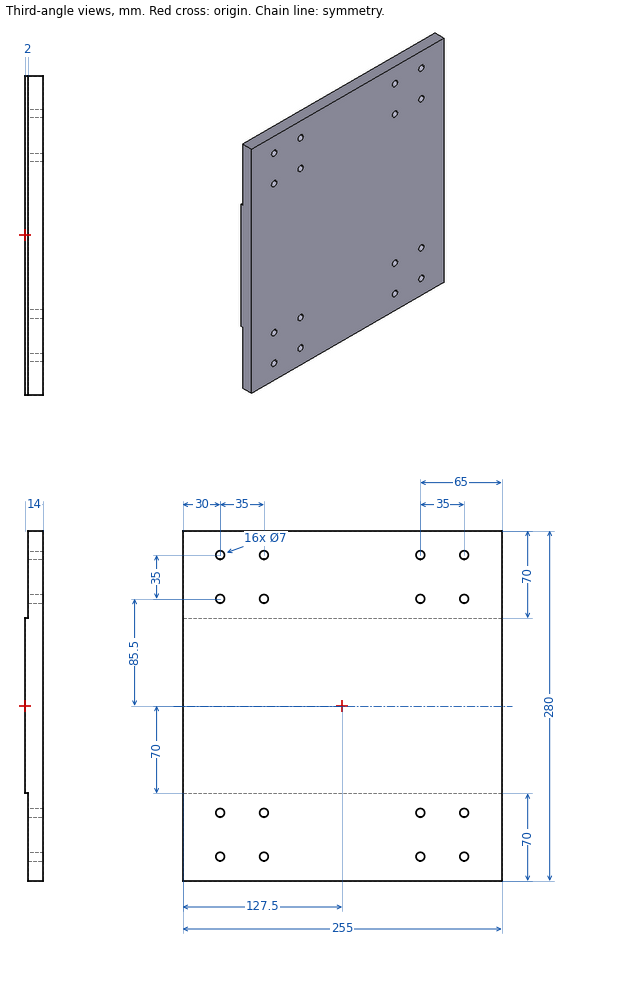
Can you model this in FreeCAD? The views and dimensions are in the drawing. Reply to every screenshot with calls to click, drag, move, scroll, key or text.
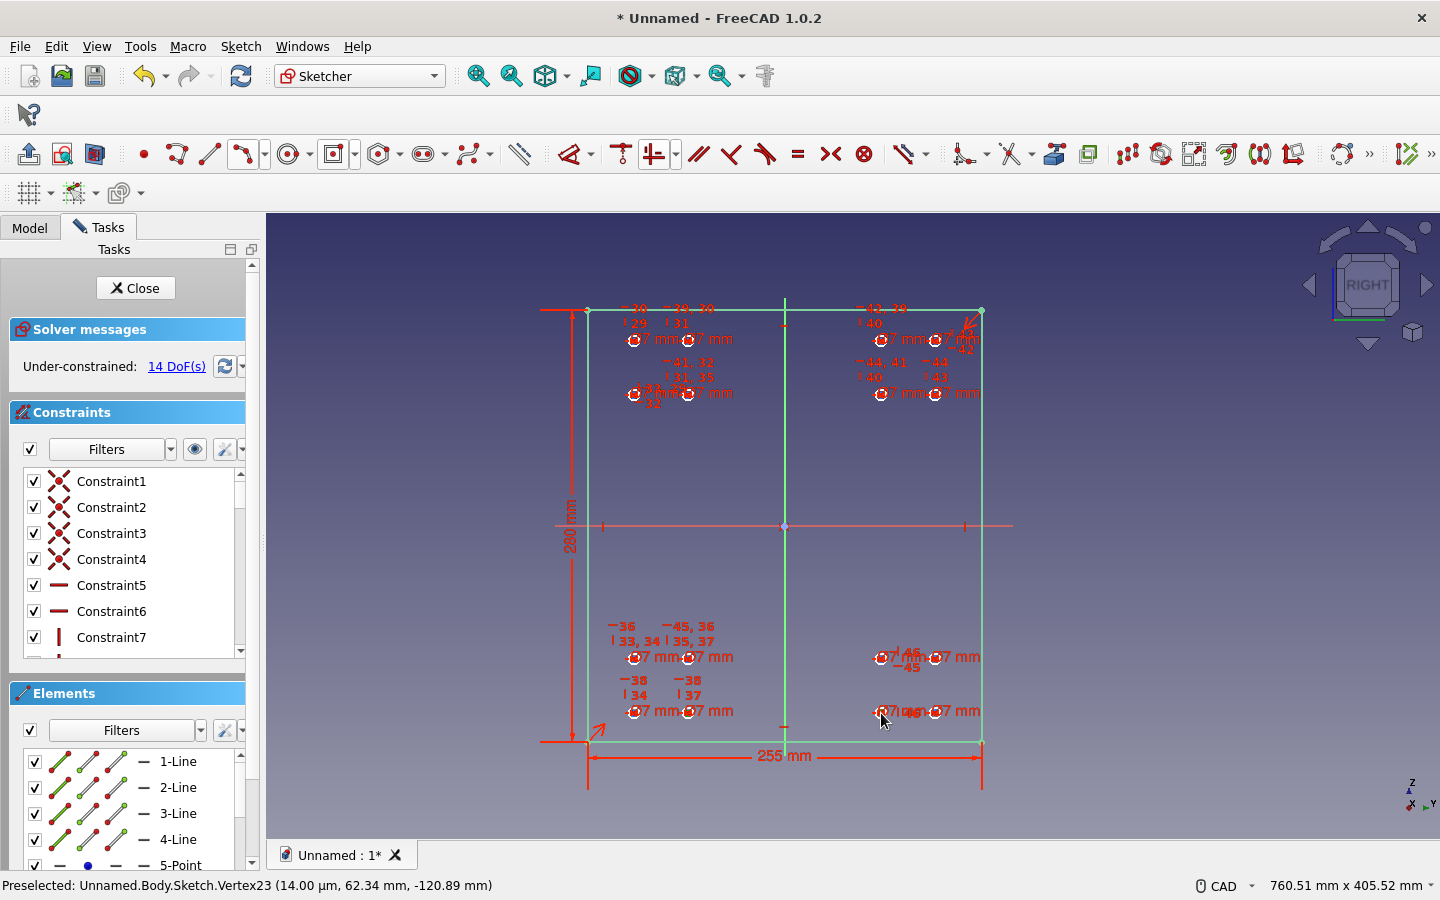
key(h)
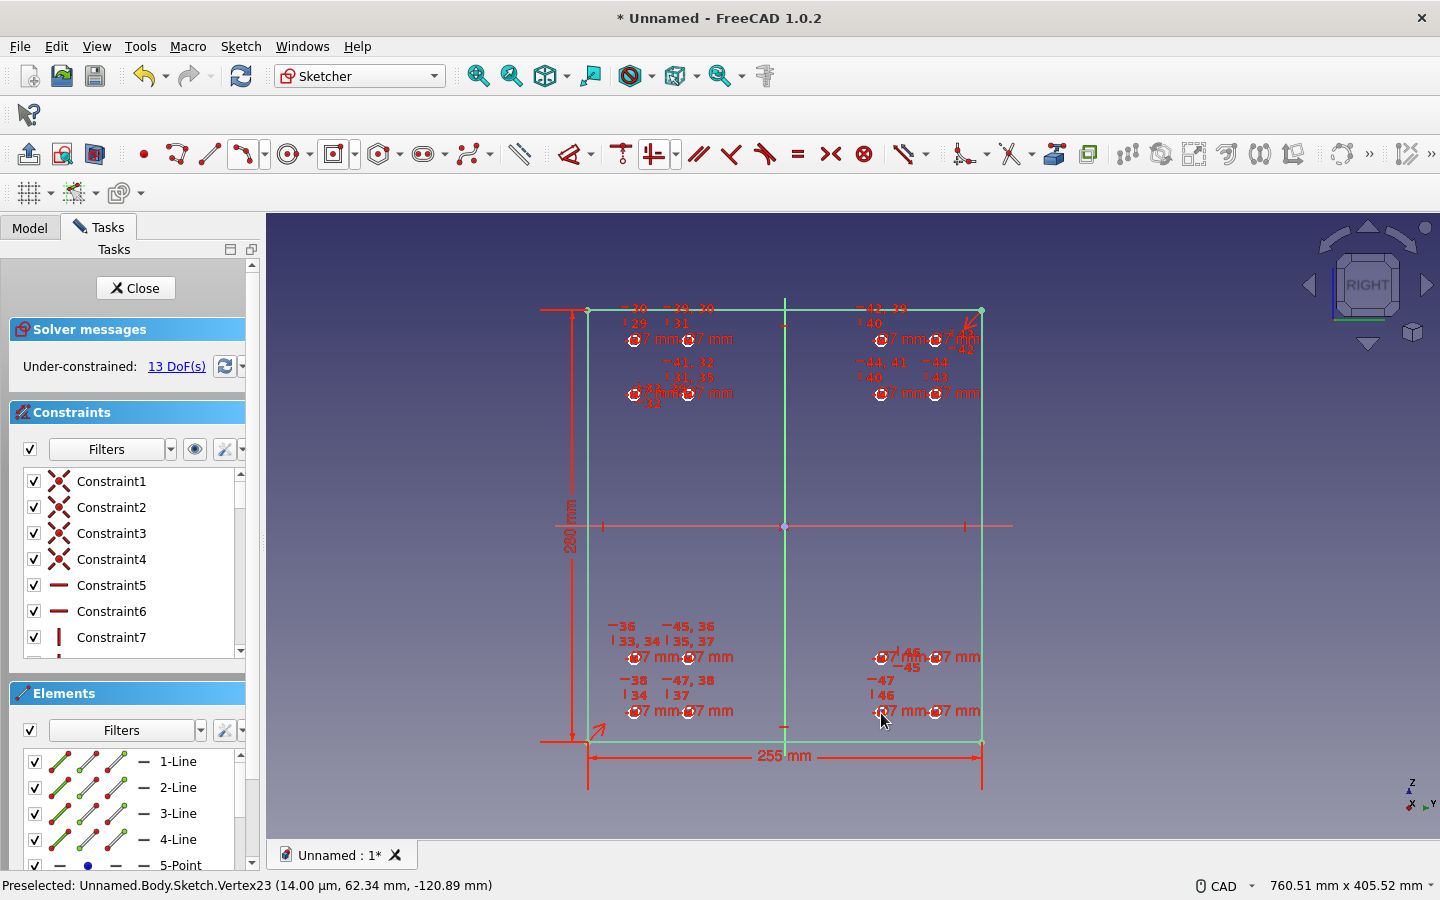
click(881, 659)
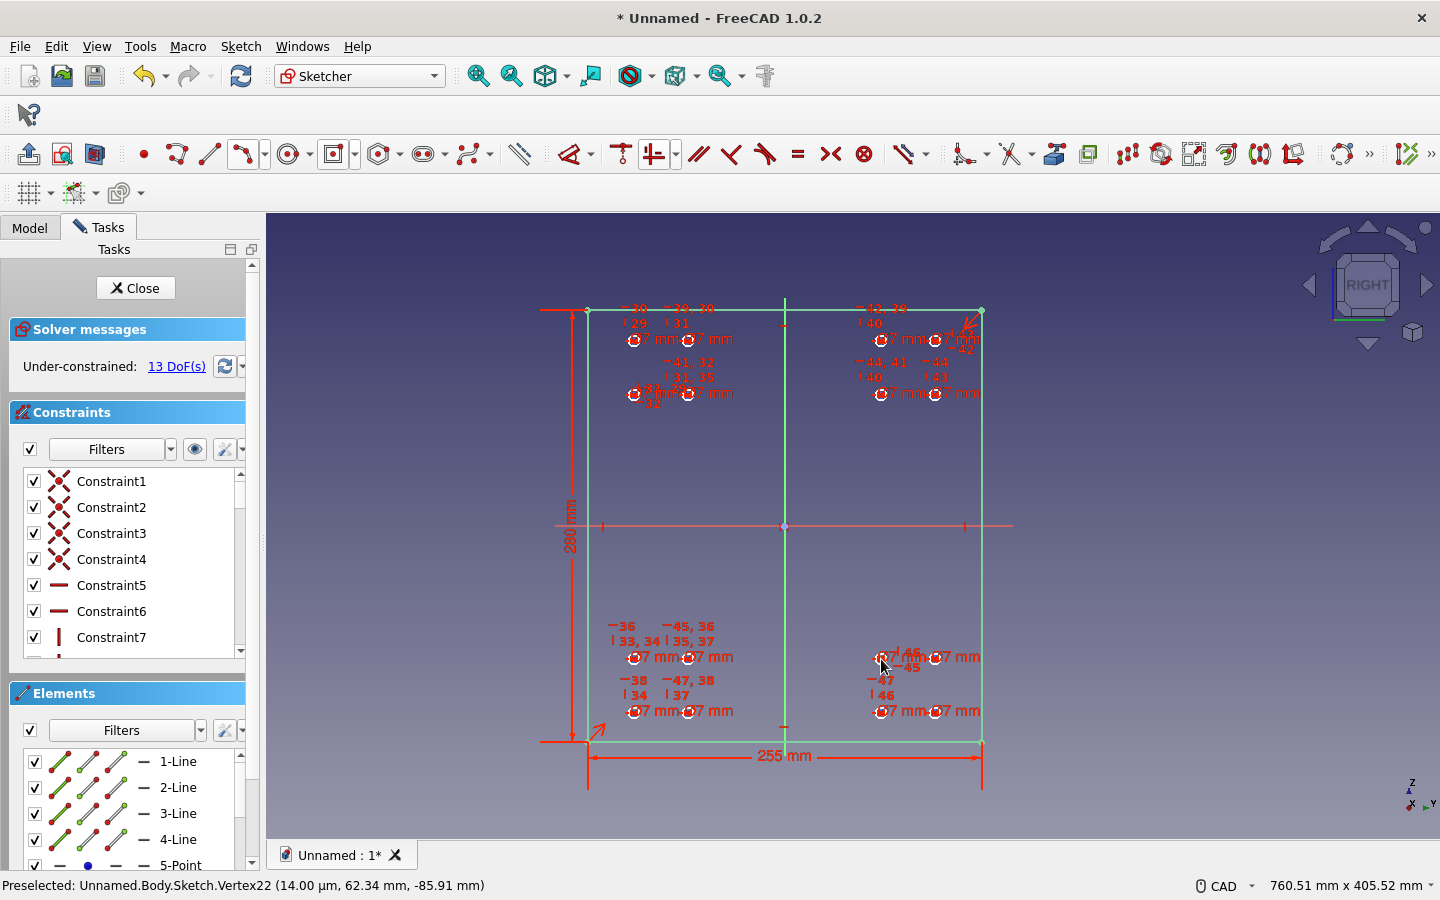
click(935, 659)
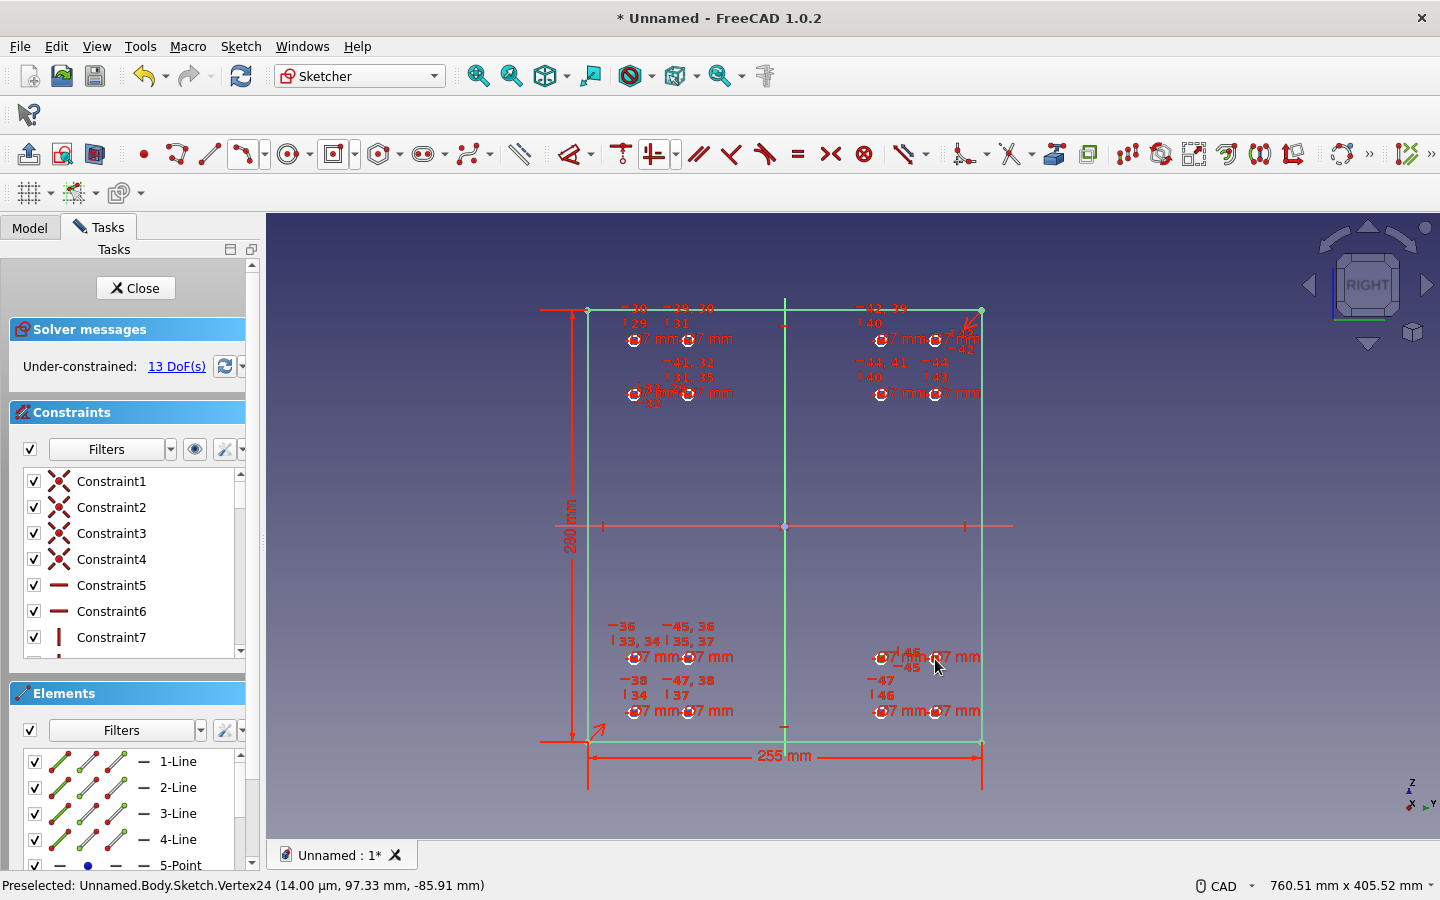
key(h)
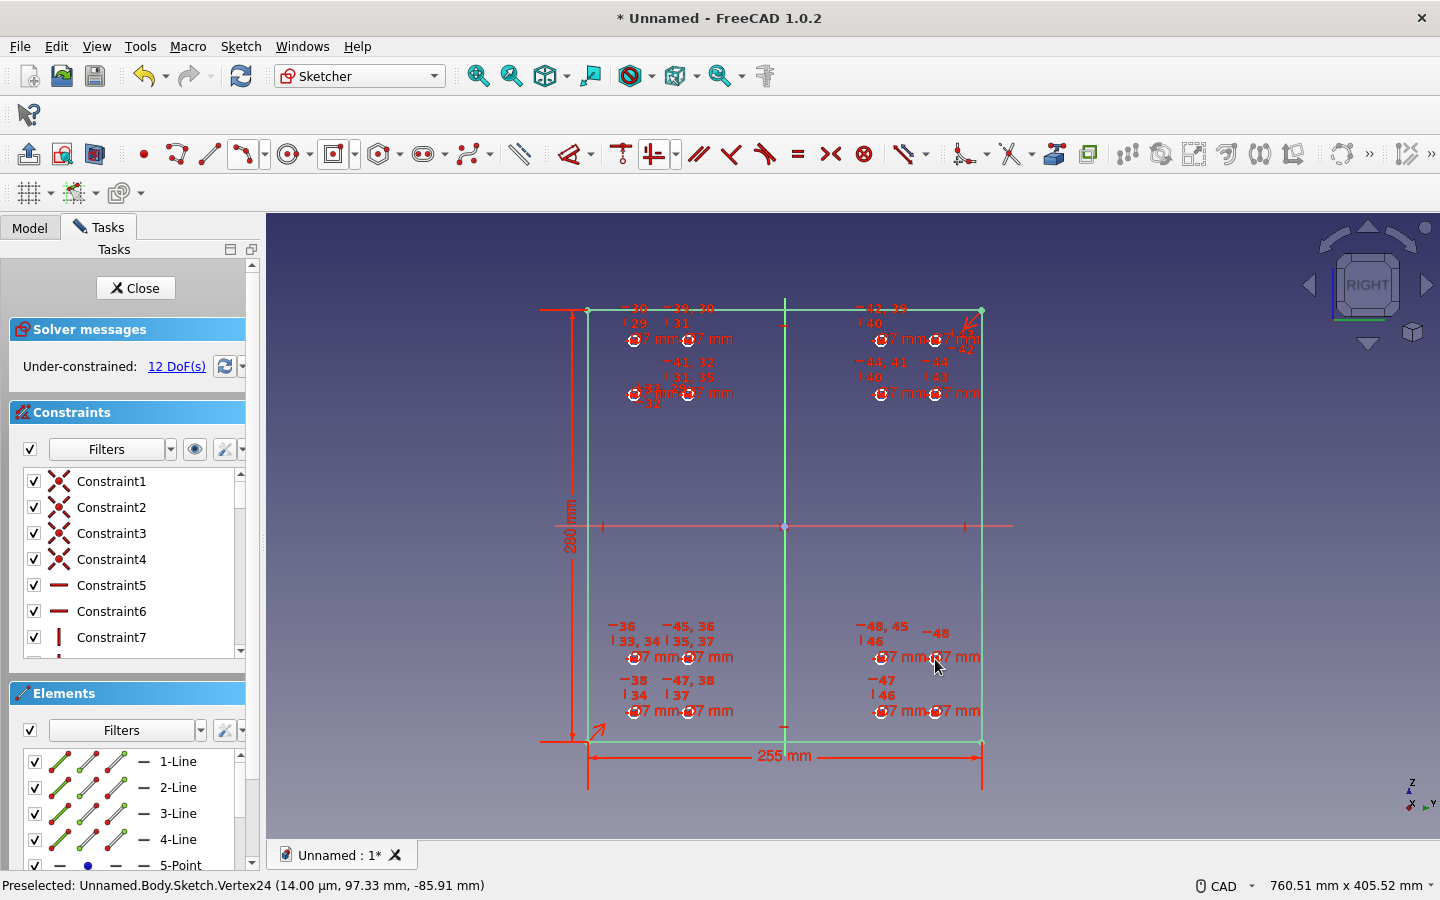
click(935, 659)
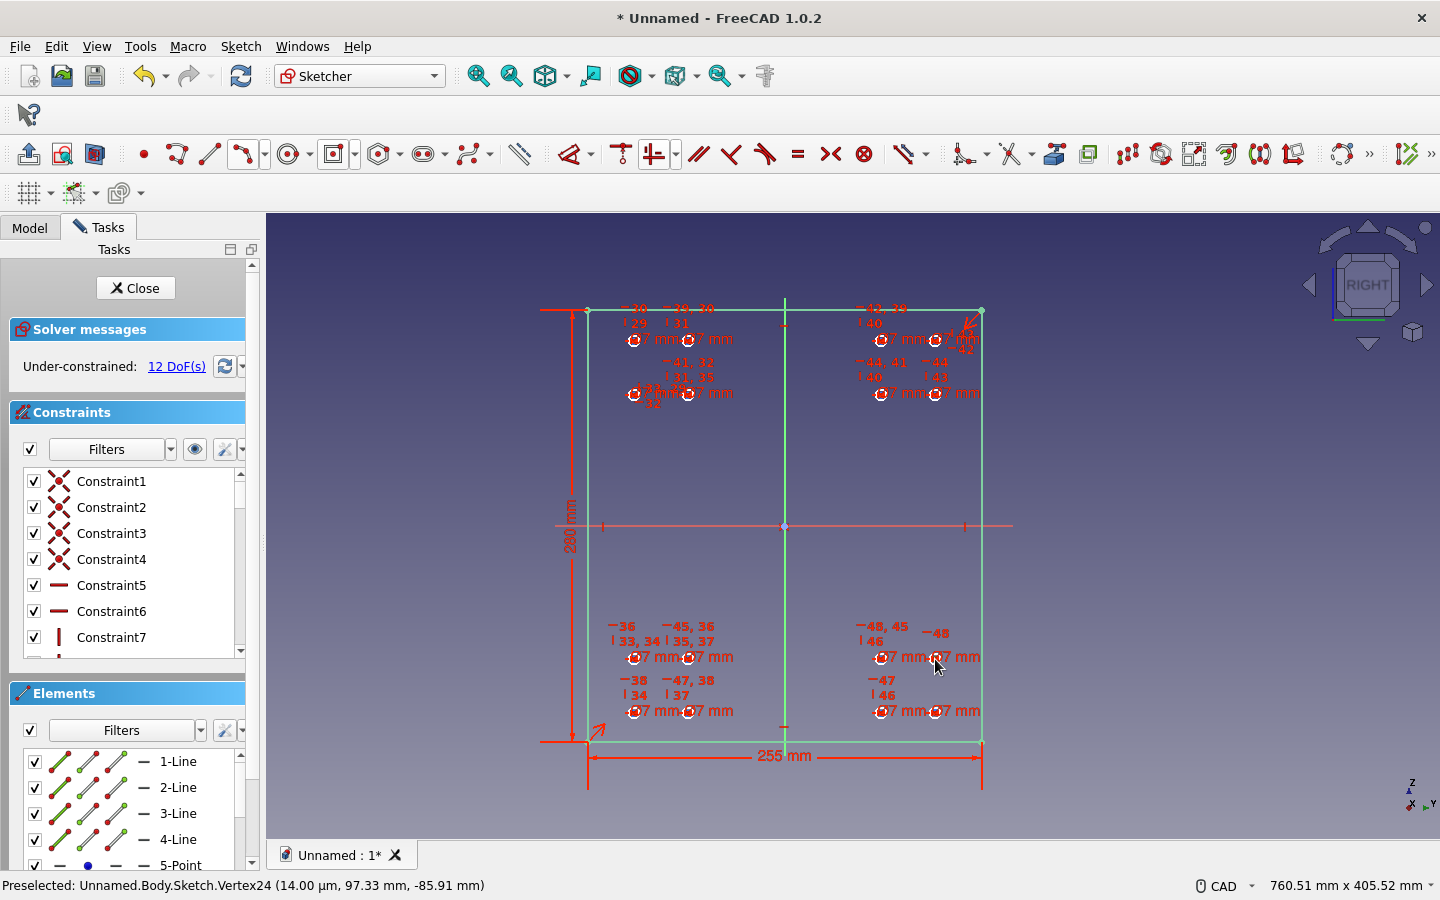
click(935, 713)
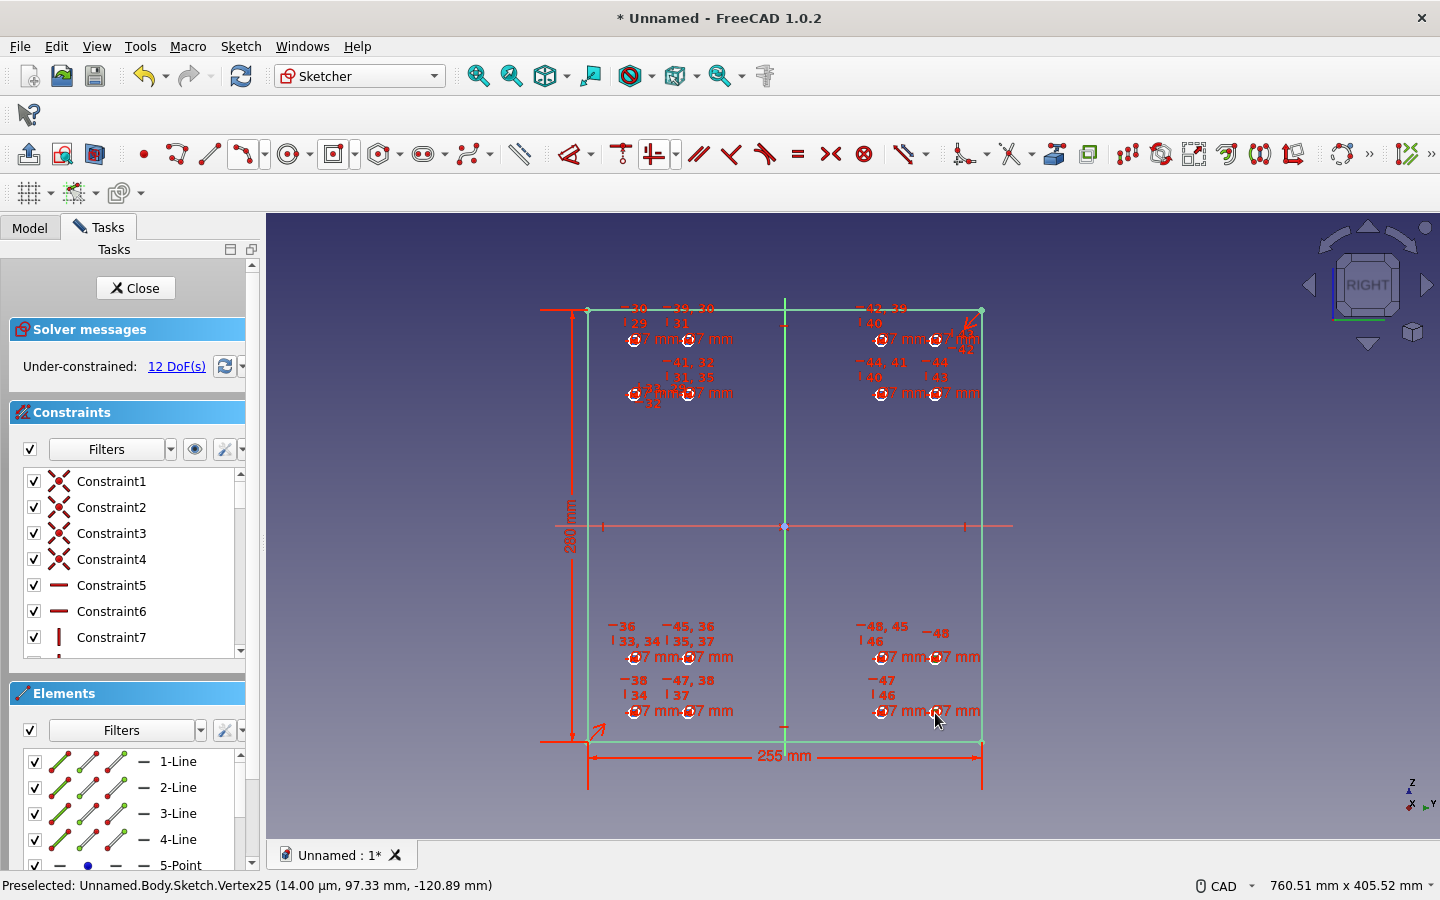
click(676, 154)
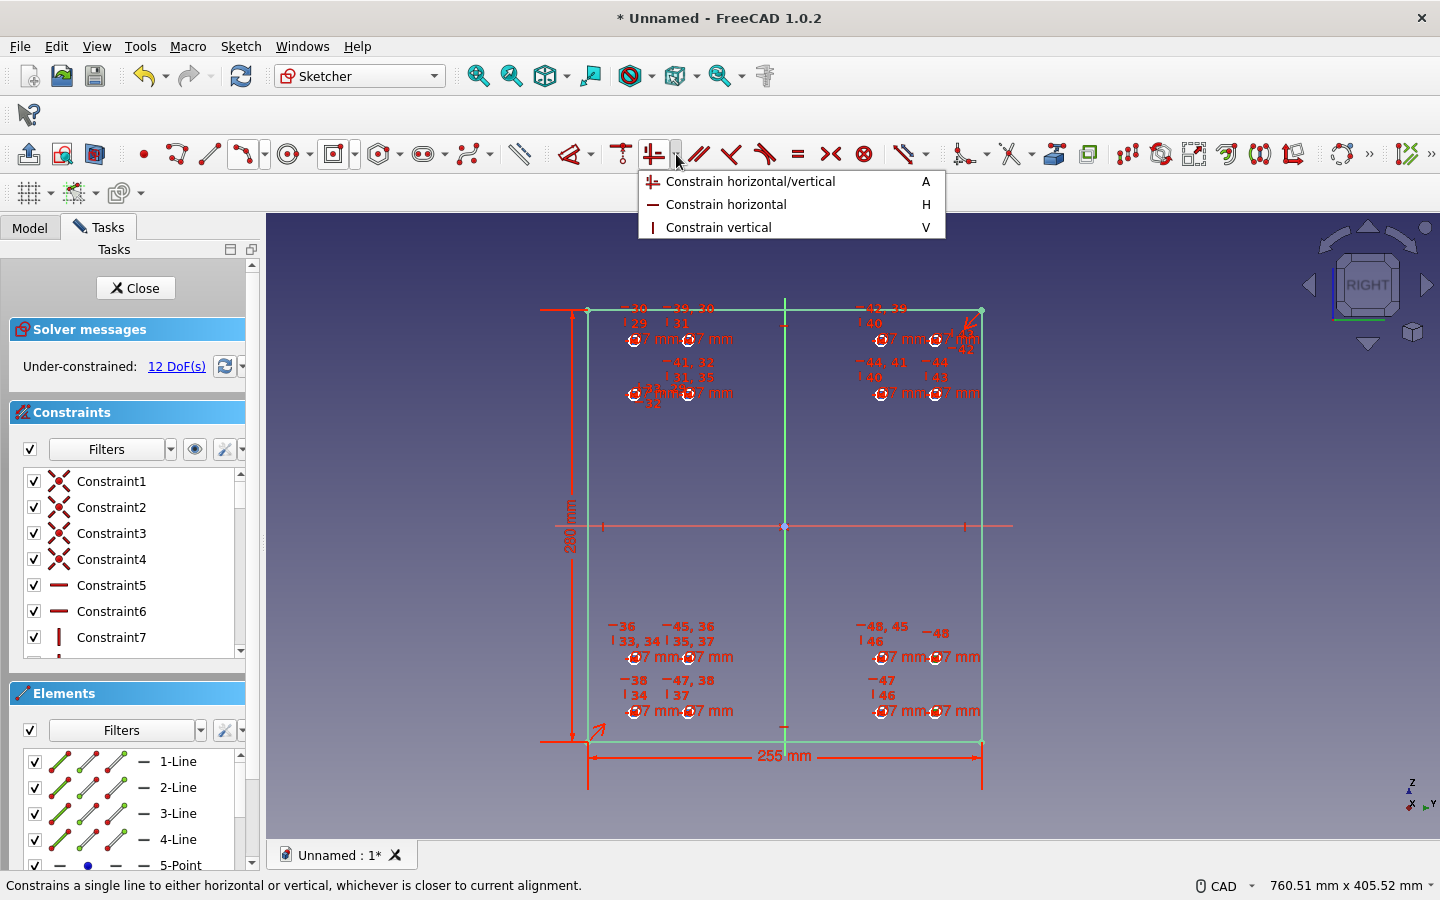
click(792, 228)